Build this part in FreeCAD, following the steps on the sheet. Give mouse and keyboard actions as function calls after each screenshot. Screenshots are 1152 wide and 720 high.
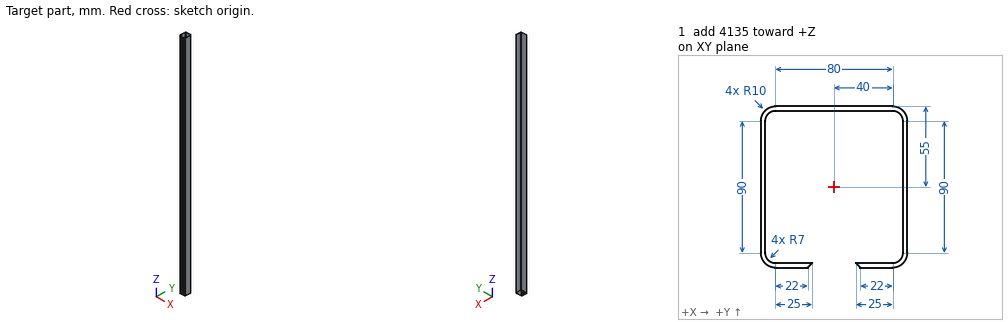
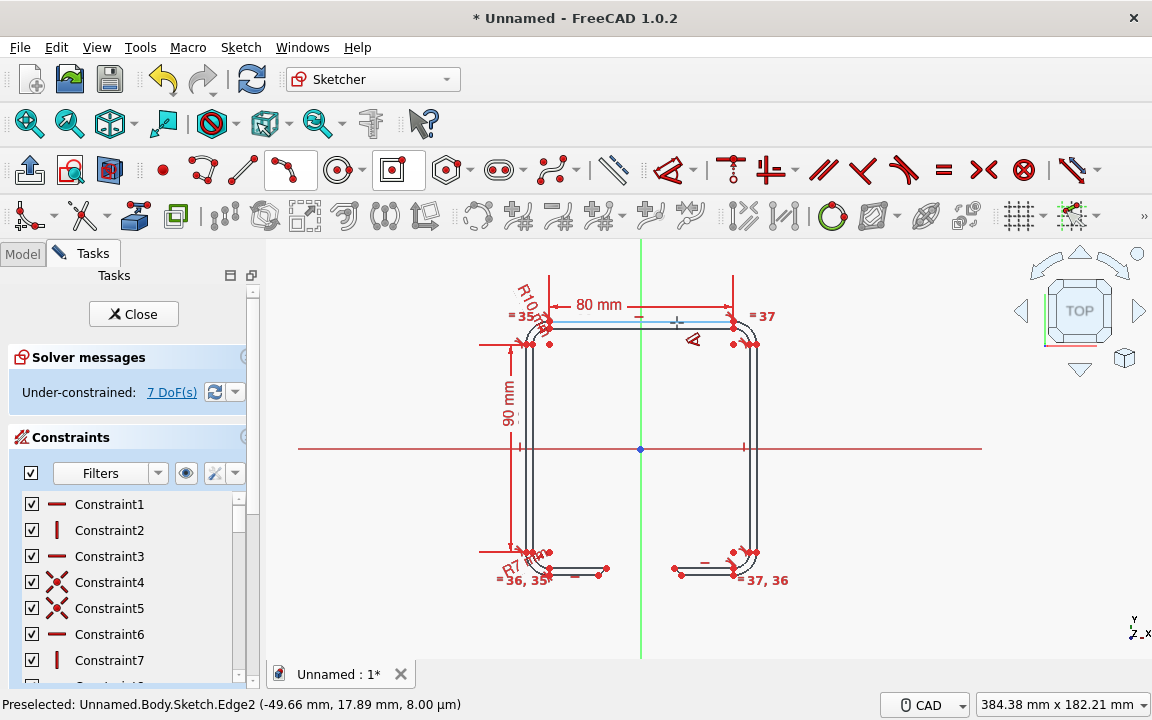
scroll(564, 575, up, 4)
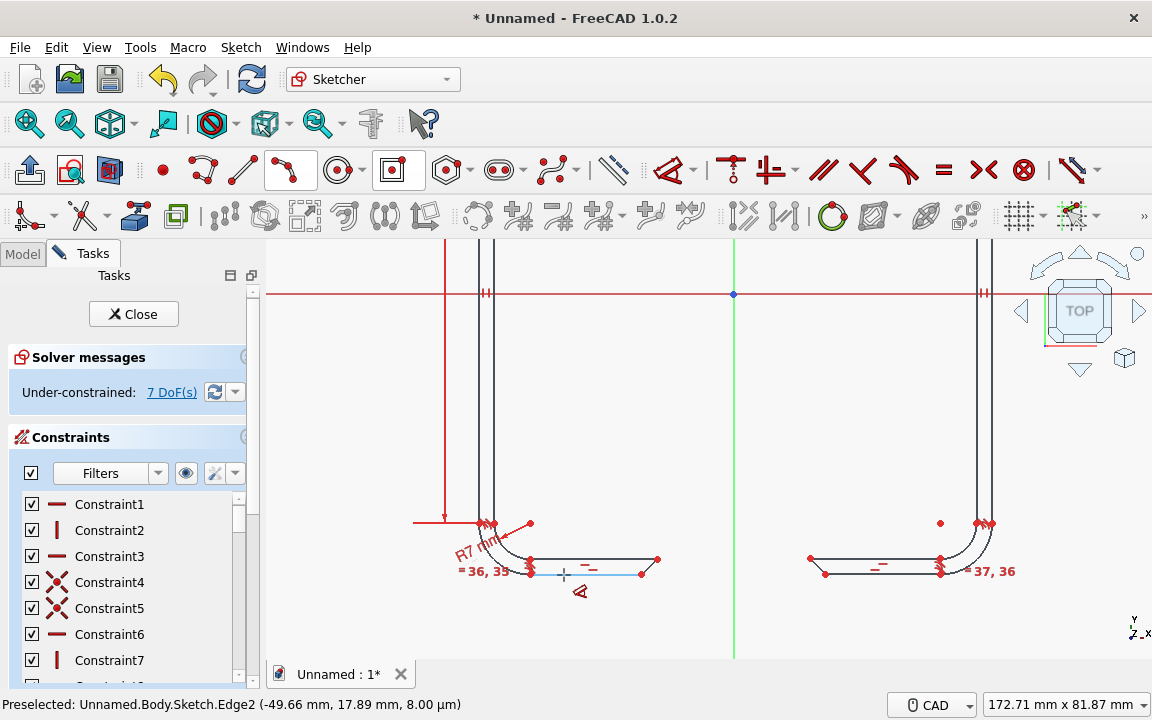
click(564, 575)
click(586, 609)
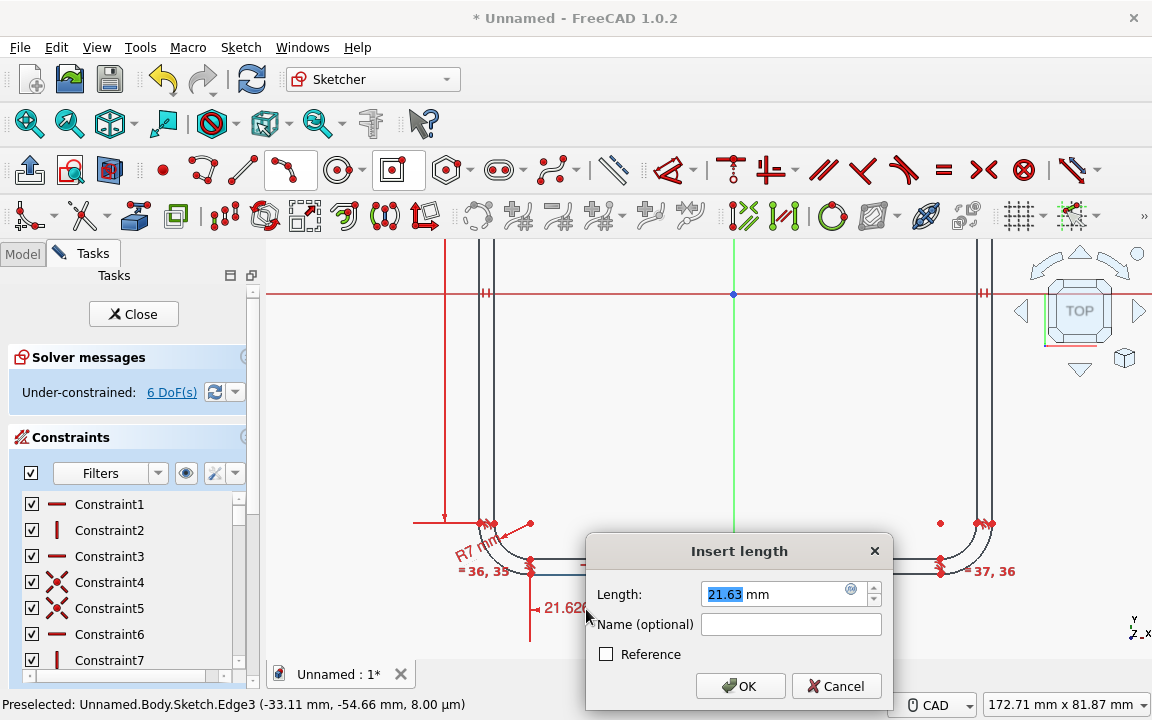
text(22)
key(Return)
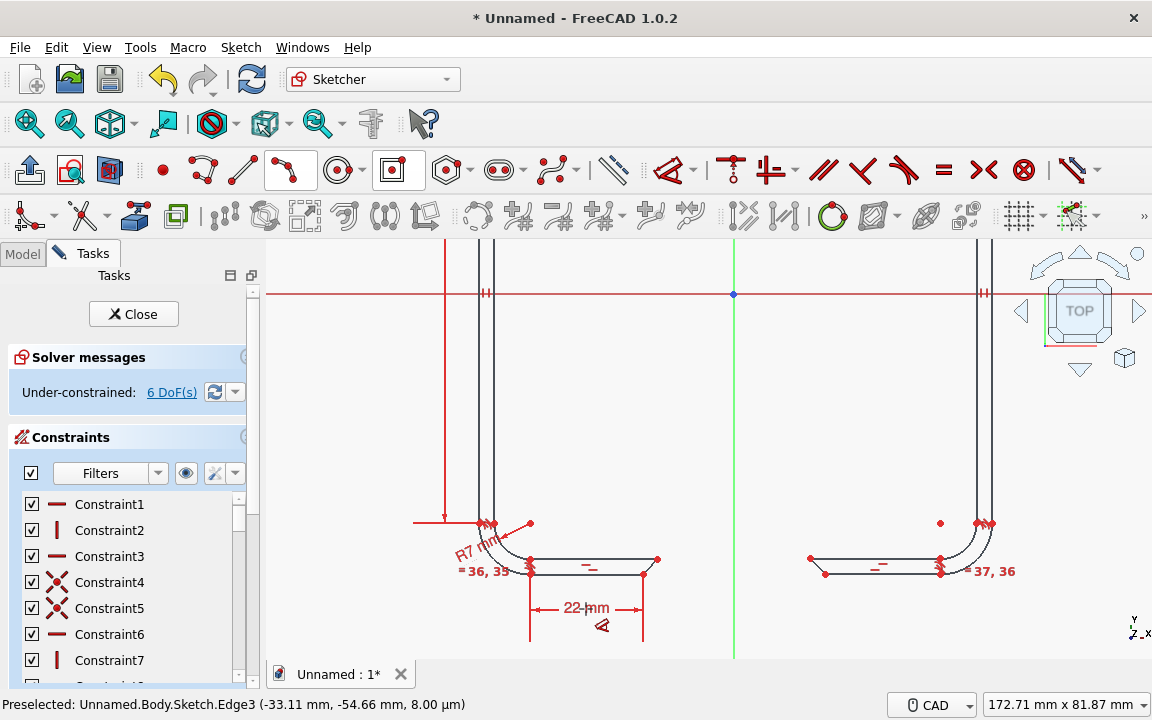
click(619, 559)
click(594, 525)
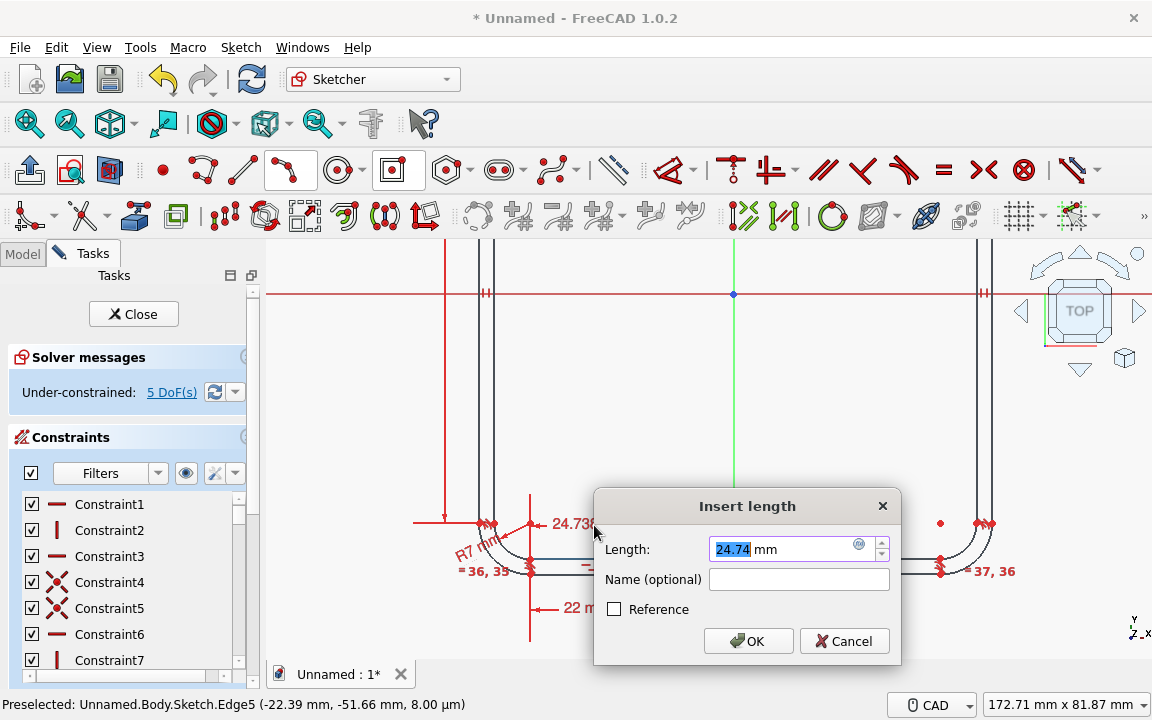
text(25)
key(Return)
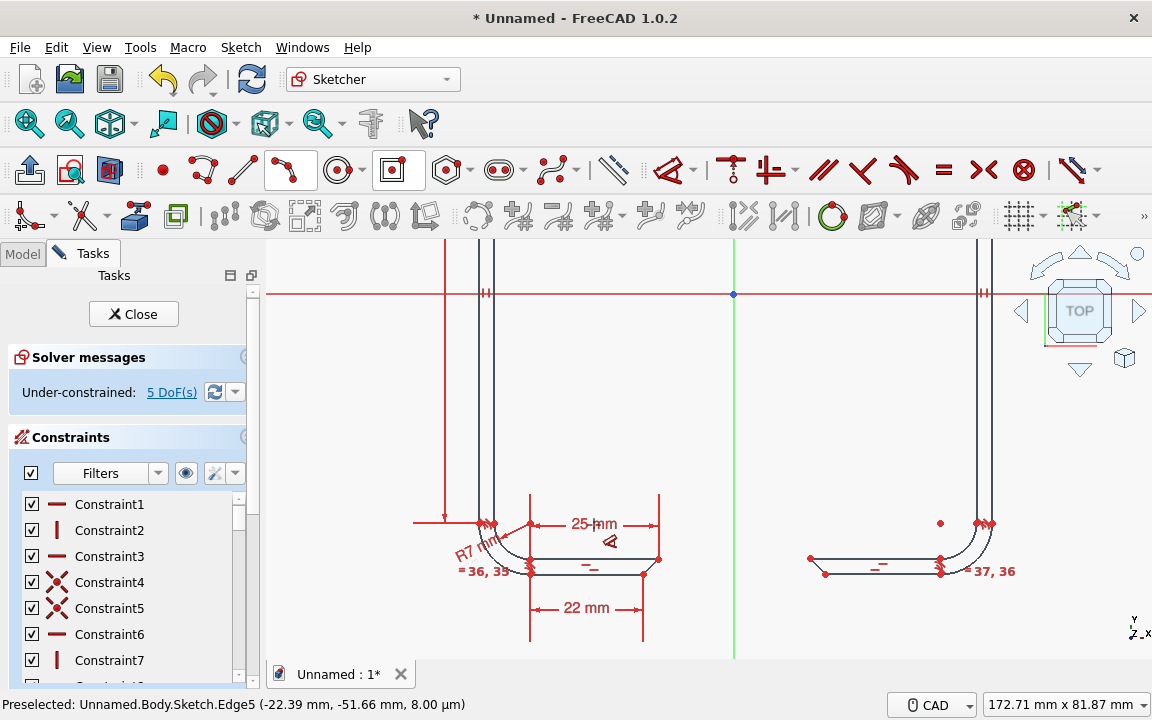
click(977, 385)
click(943, 395)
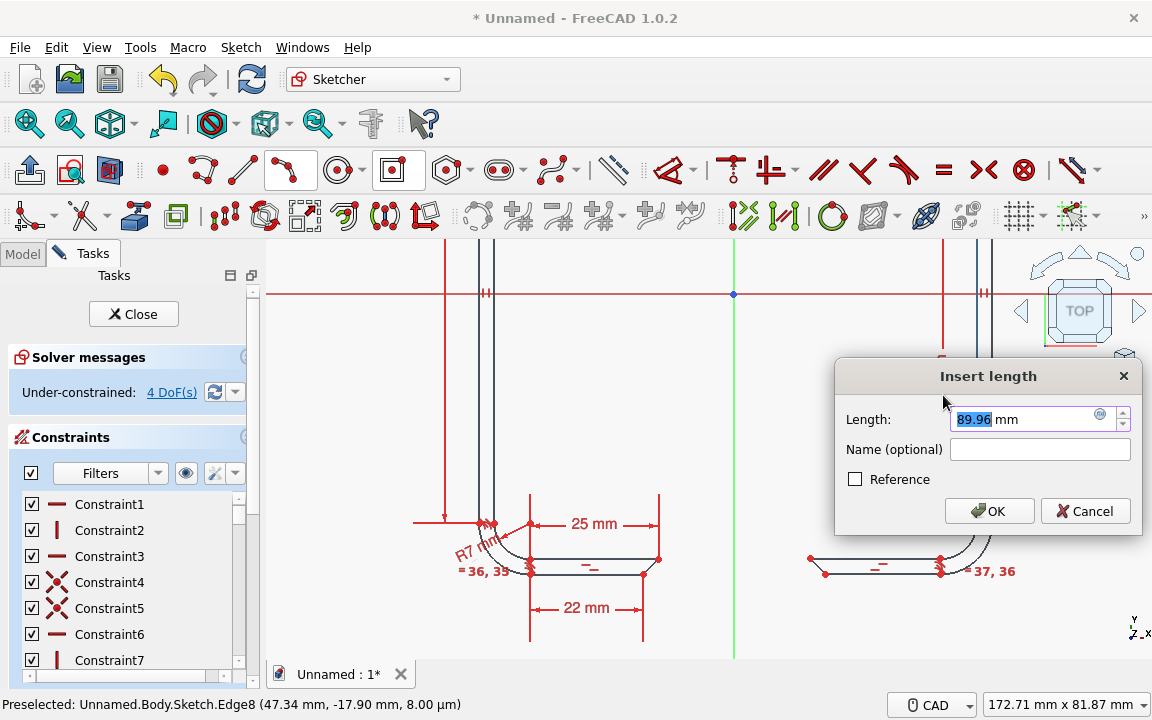
text(90)
key(Return)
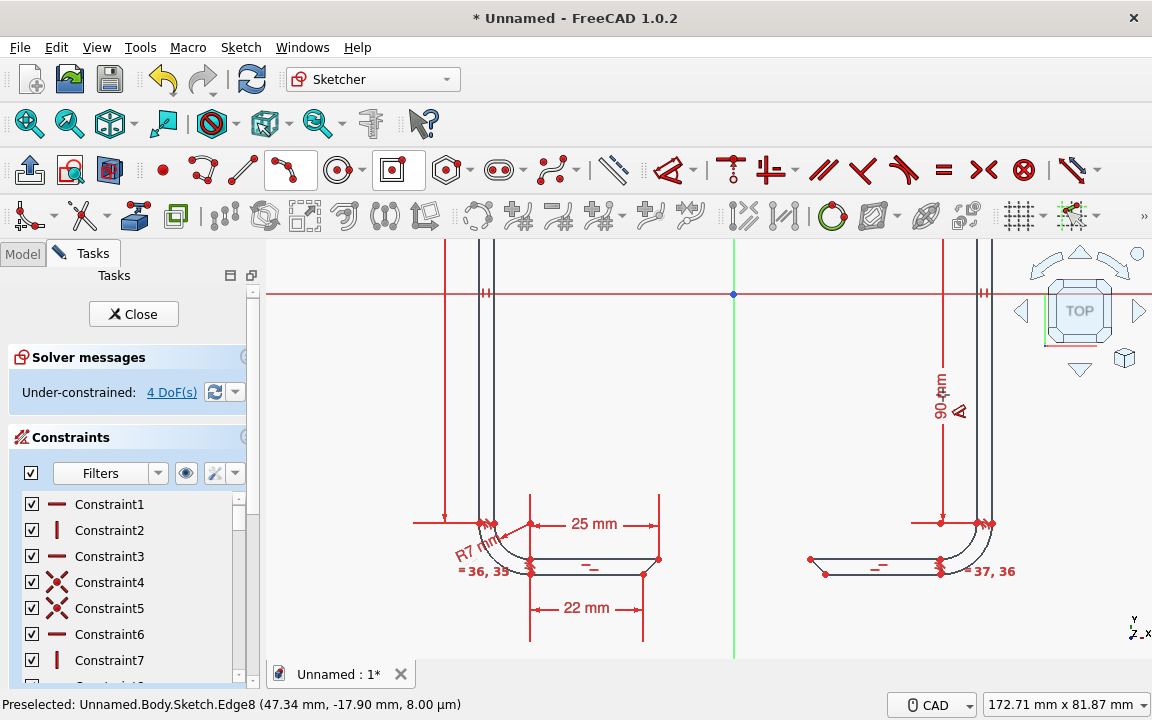
click(902, 559)
click(876, 593)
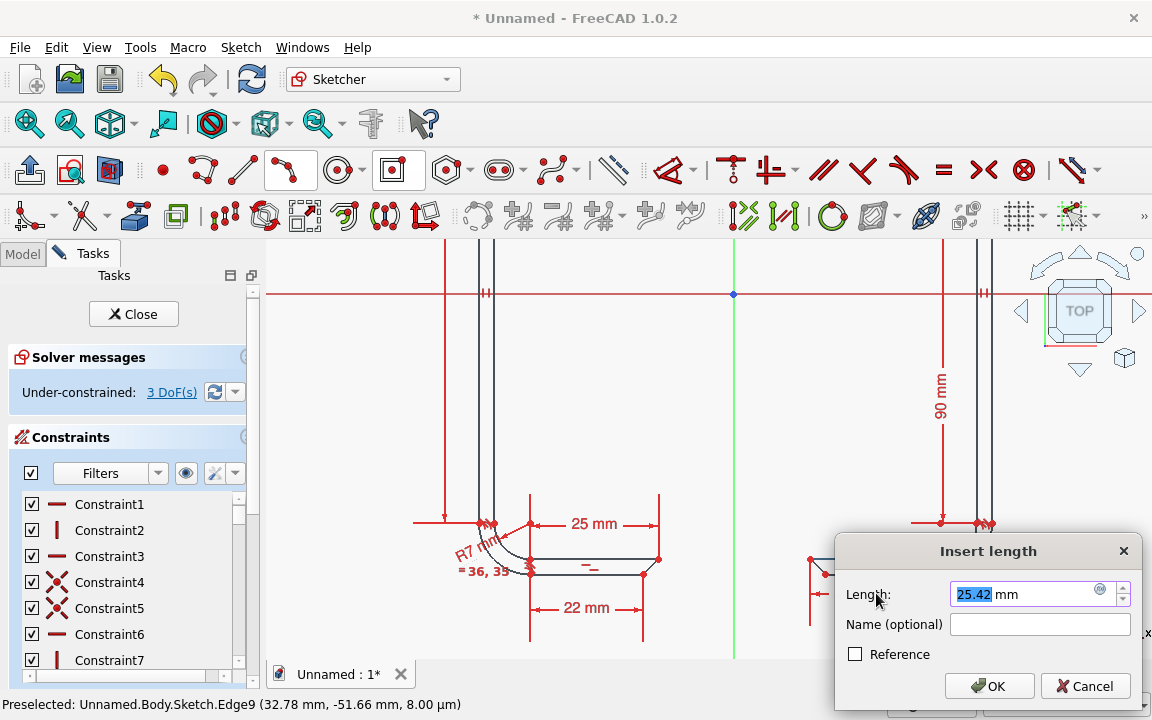
text(25)
key(Return)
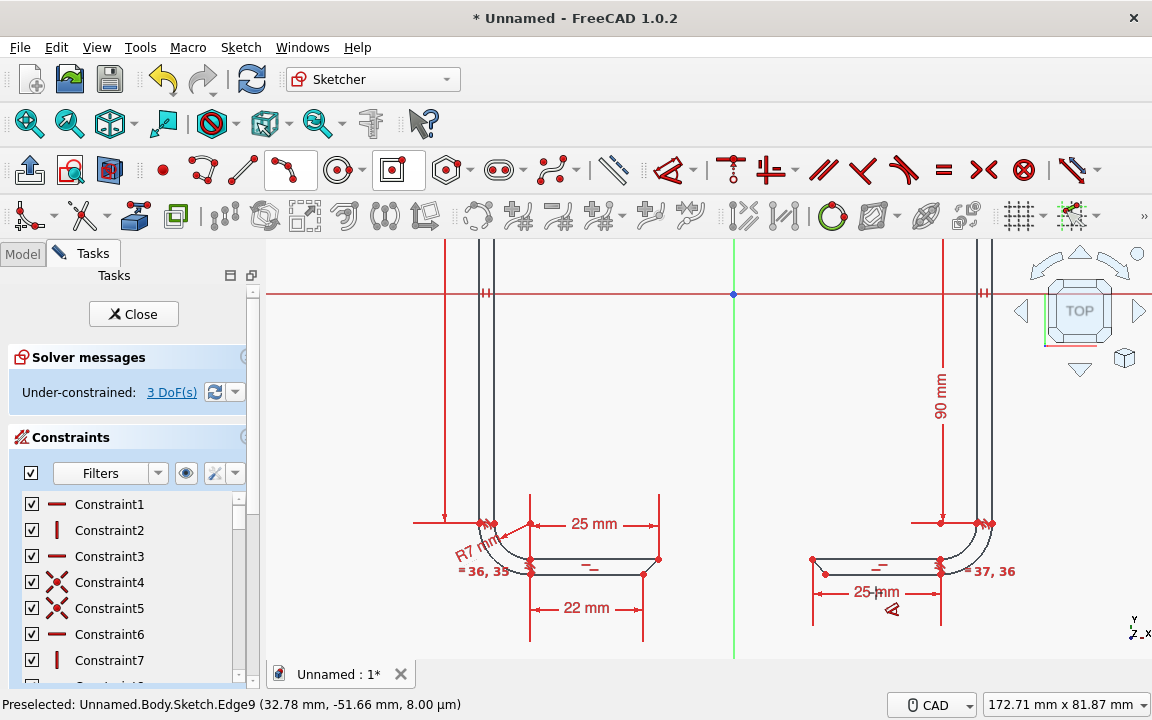
click(860, 575)
click(883, 541)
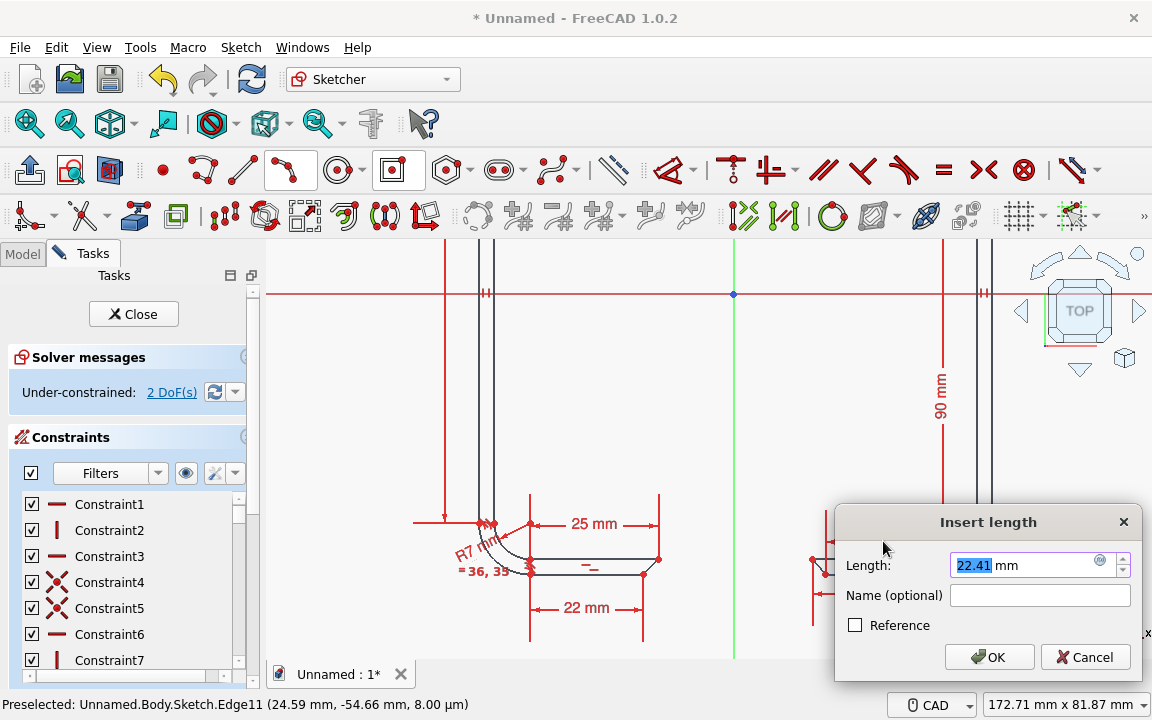
text(22)
key(Return)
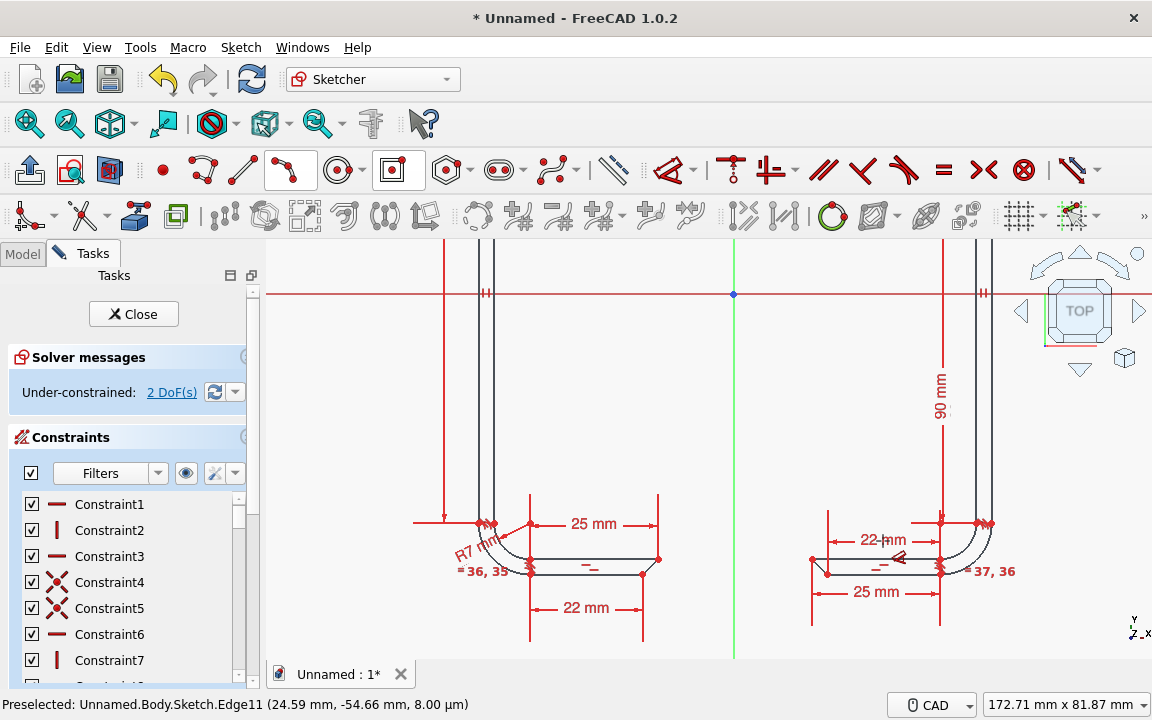
scroll(564, 575, down, 4)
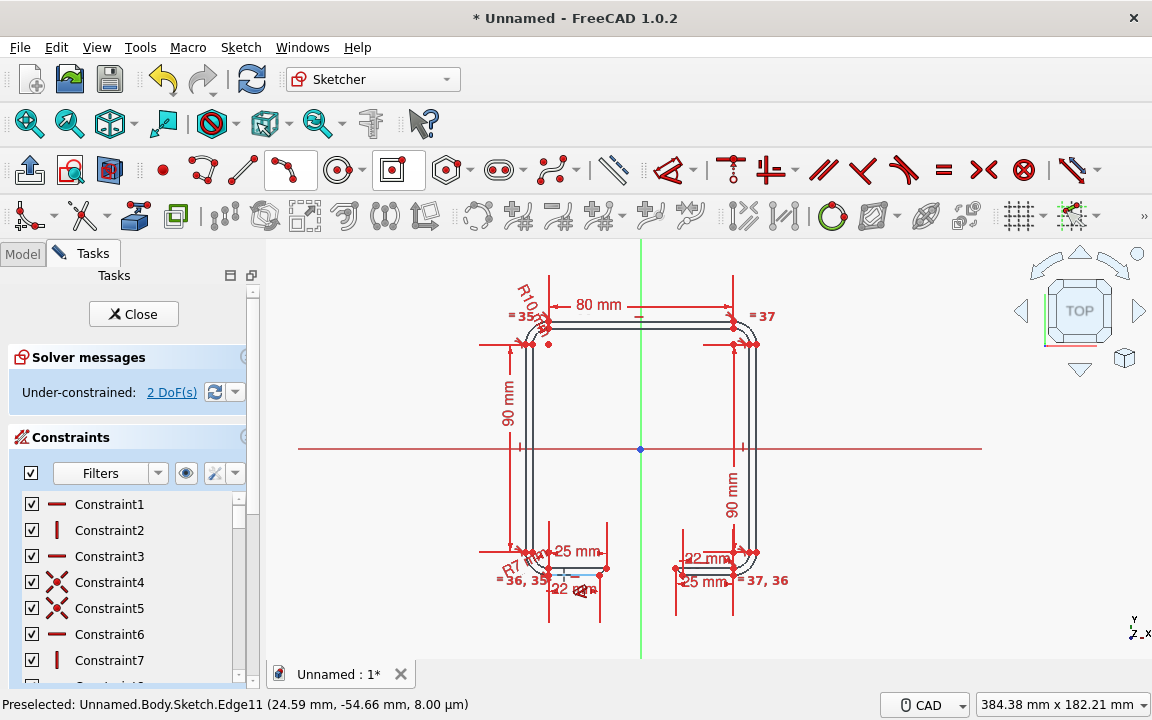
scroll(733, 322, up, 3)